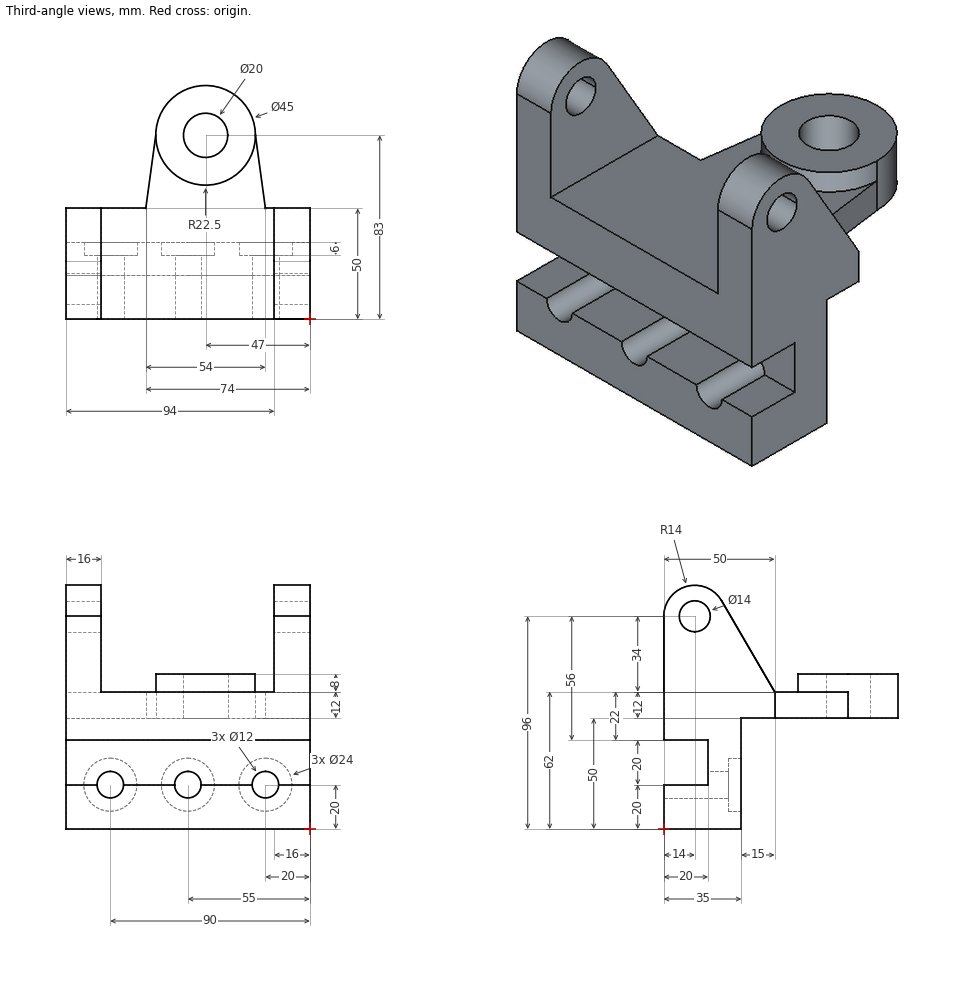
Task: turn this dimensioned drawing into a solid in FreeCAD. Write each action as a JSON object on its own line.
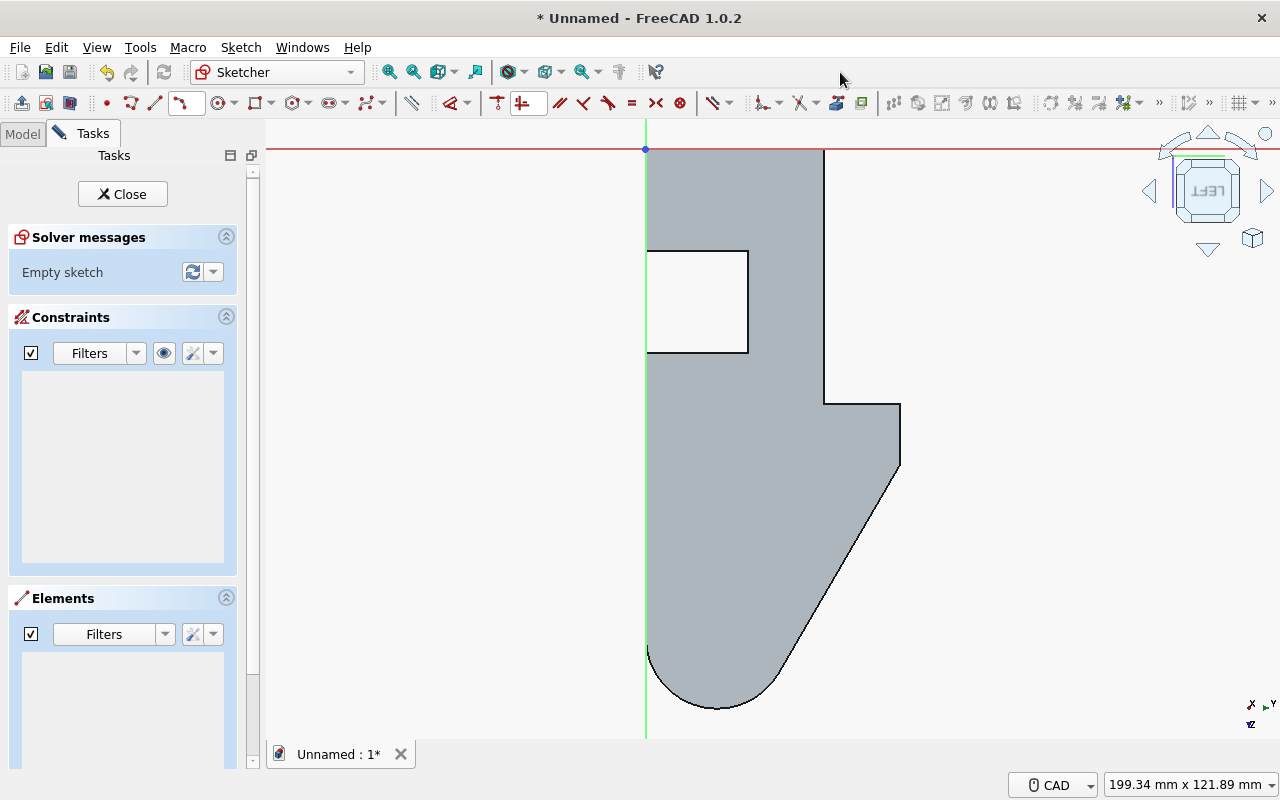
{"action": "scroll", "coordinate": [395, 711], "scroll_direction": "down", "scroll_amount": 1}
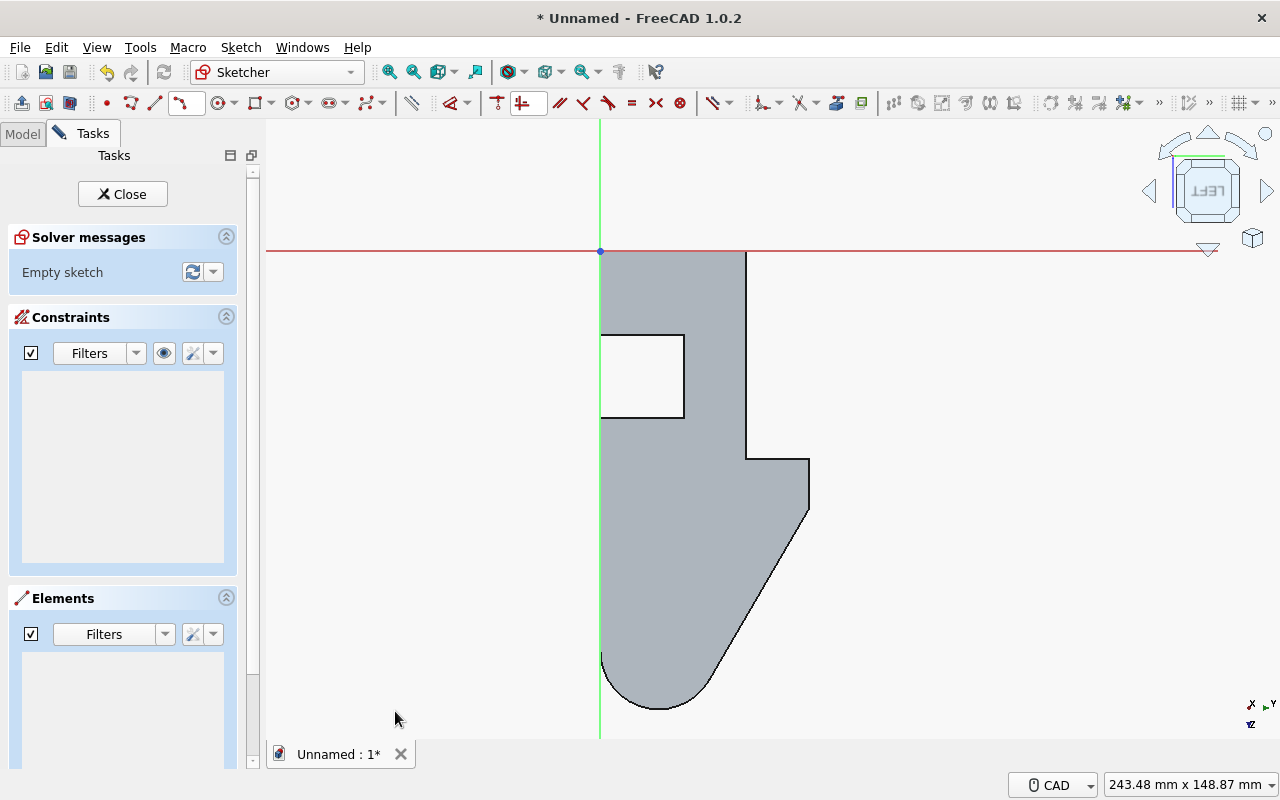
{"action": "scroll", "coordinate": [705, 281], "scroll_direction": "up", "scroll_amount": 2}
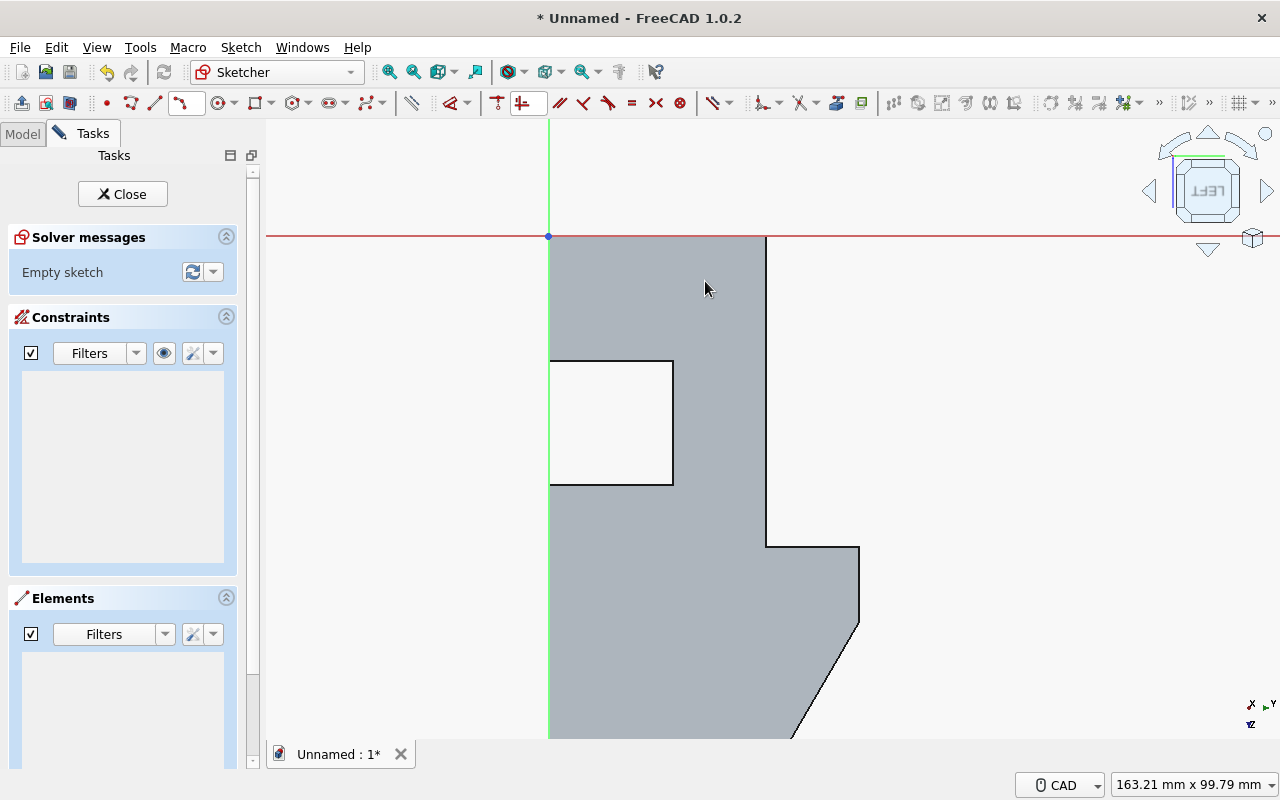
{"action": "key", "text": "g m"}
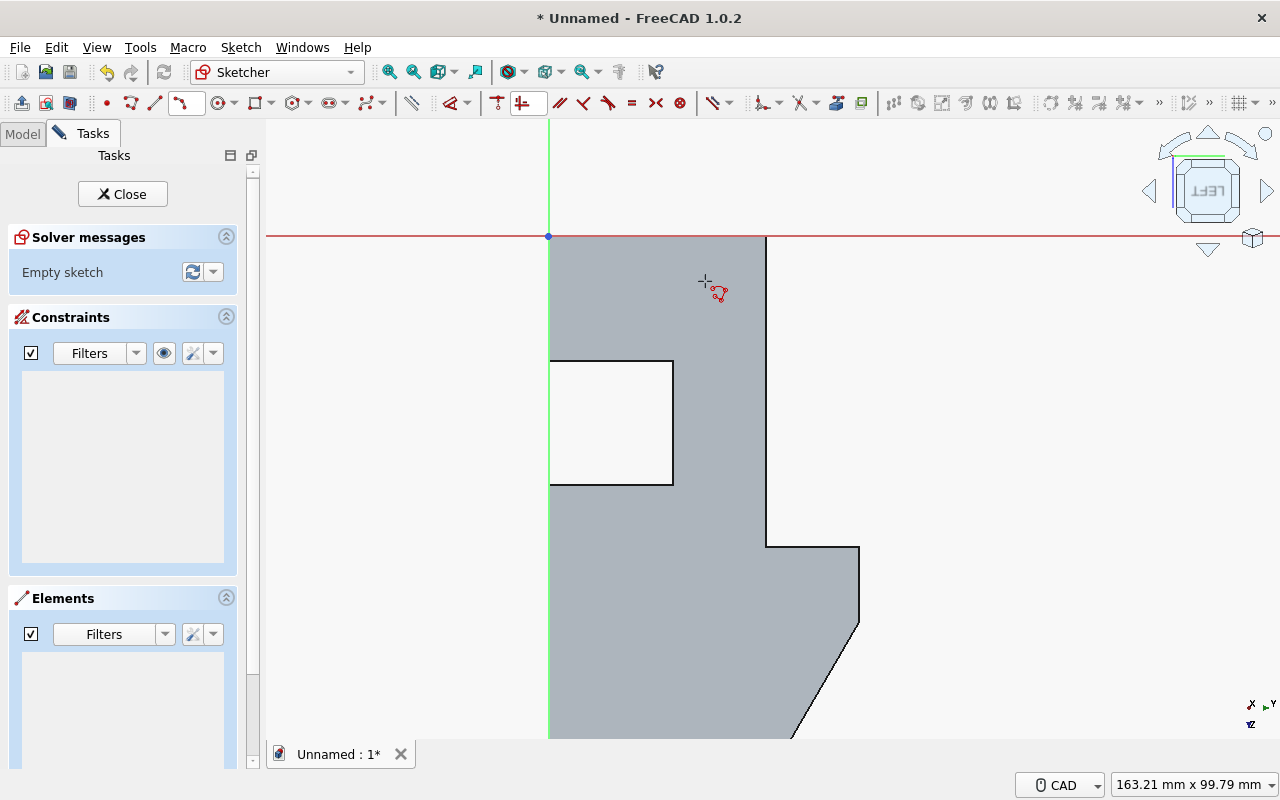
{"action": "left_click", "coordinate": [549, 236]}
{"action": "left_click", "coordinate": [558, 361]}
{"action": "left_click", "coordinate": [673, 361]}
{"action": "left_click", "coordinate": [673, 485]}
{"action": "left_click", "coordinate": [549, 485]}
{"action": "left_click", "coordinate": [558, 622]}
{"action": "left_click", "coordinate": [859, 622]}
{"action": "left_click", "coordinate": [859, 547]}
{"action": "left_click", "coordinate": [766, 547]}
{"action": "left_click", "coordinate": [766, 245]}
{"action": "left_click", "coordinate": [549, 236]}
{"action": "key", "text": "Escape"}
{"action": "key", "text": "Escape"}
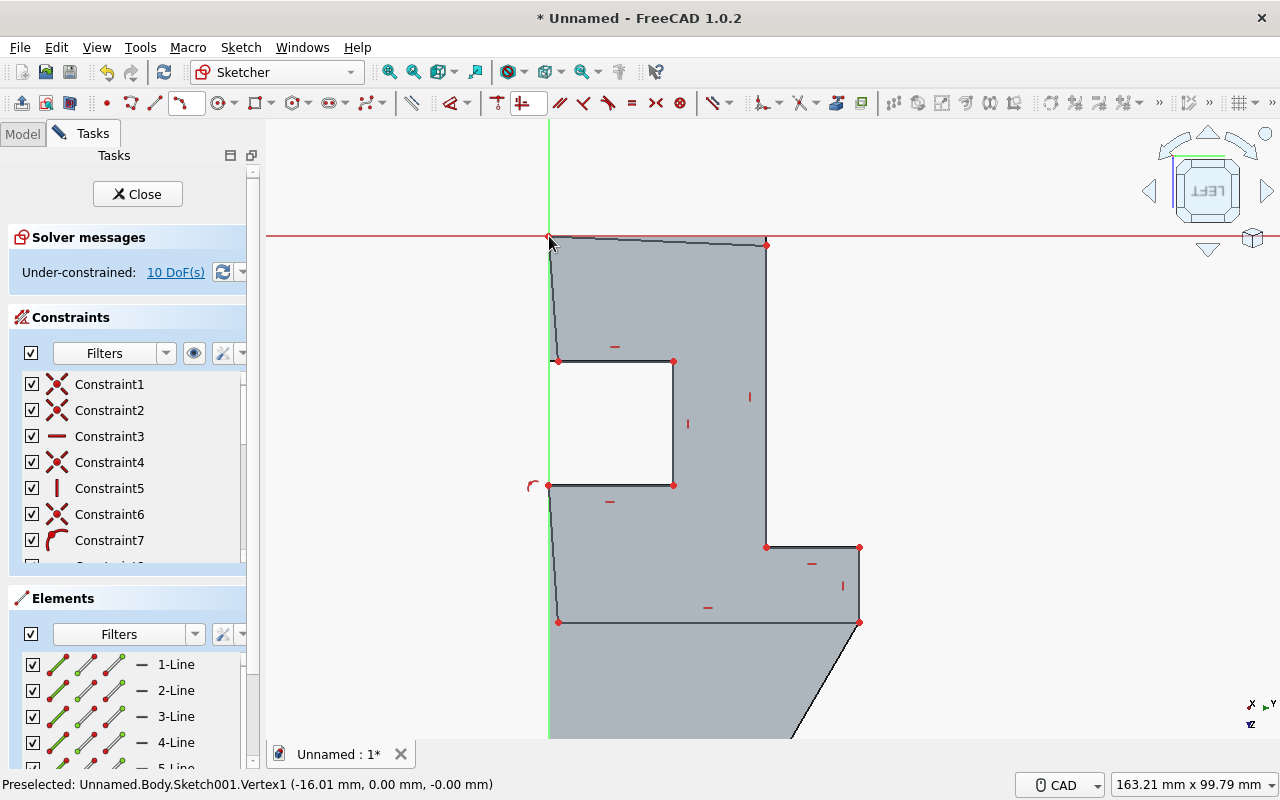
{"action": "left_click", "coordinate": [552, 274]}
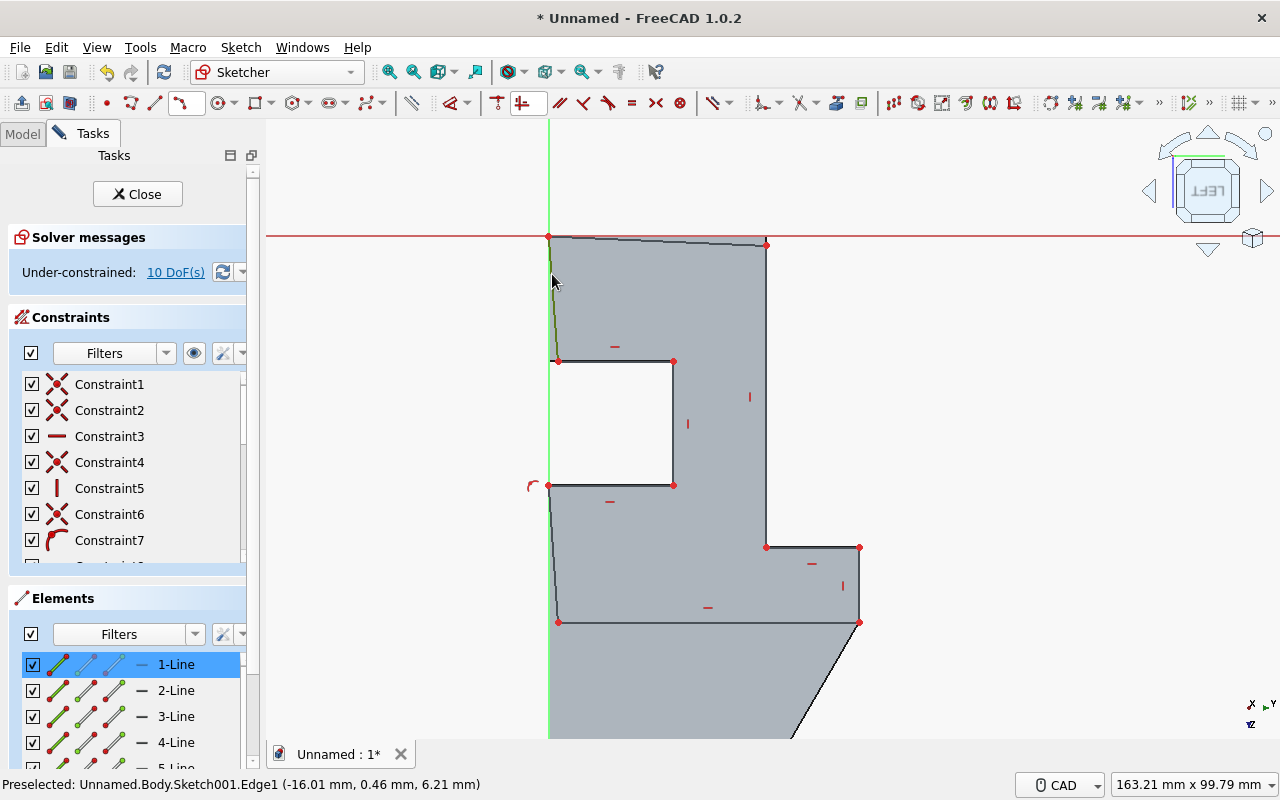
{"action": "left_click", "coordinate": [542, 104]}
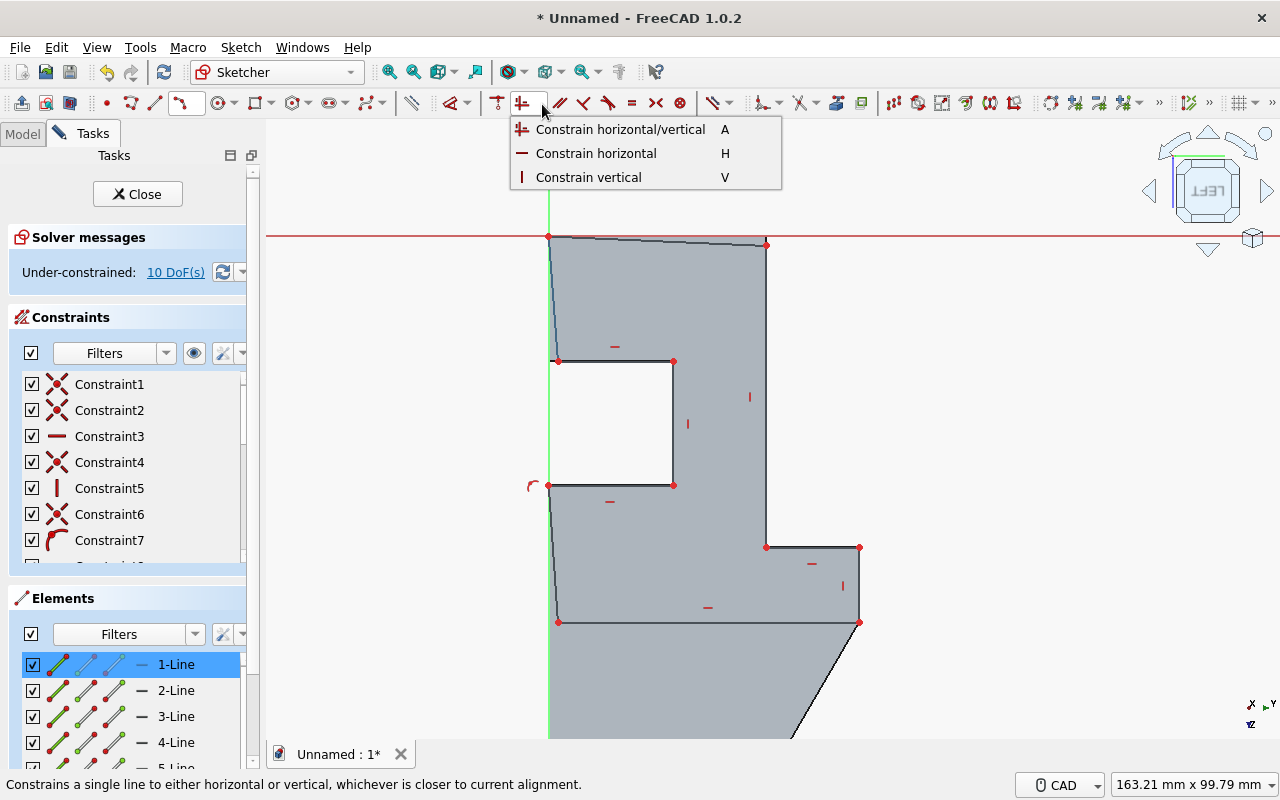
{"action": "left_click", "coordinate": [646, 177]}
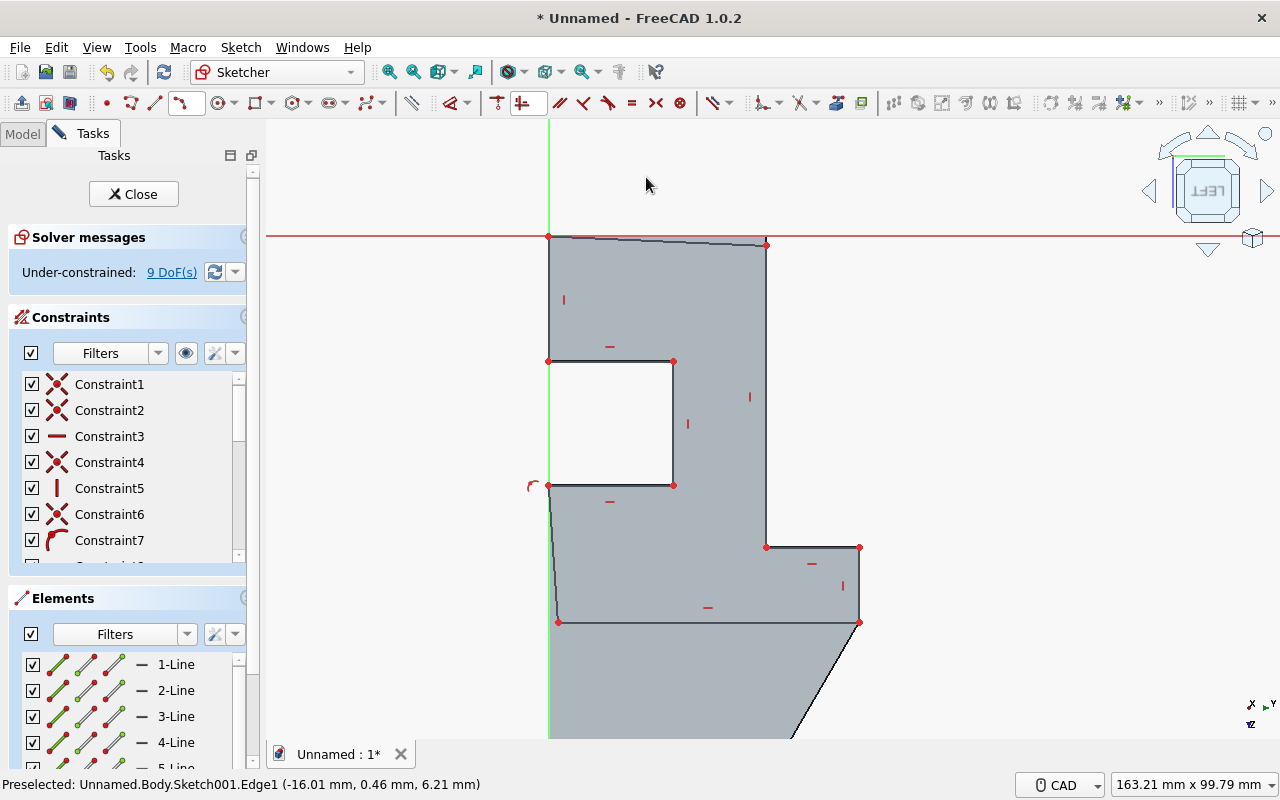
{"action": "left_click", "coordinate": [552, 527]}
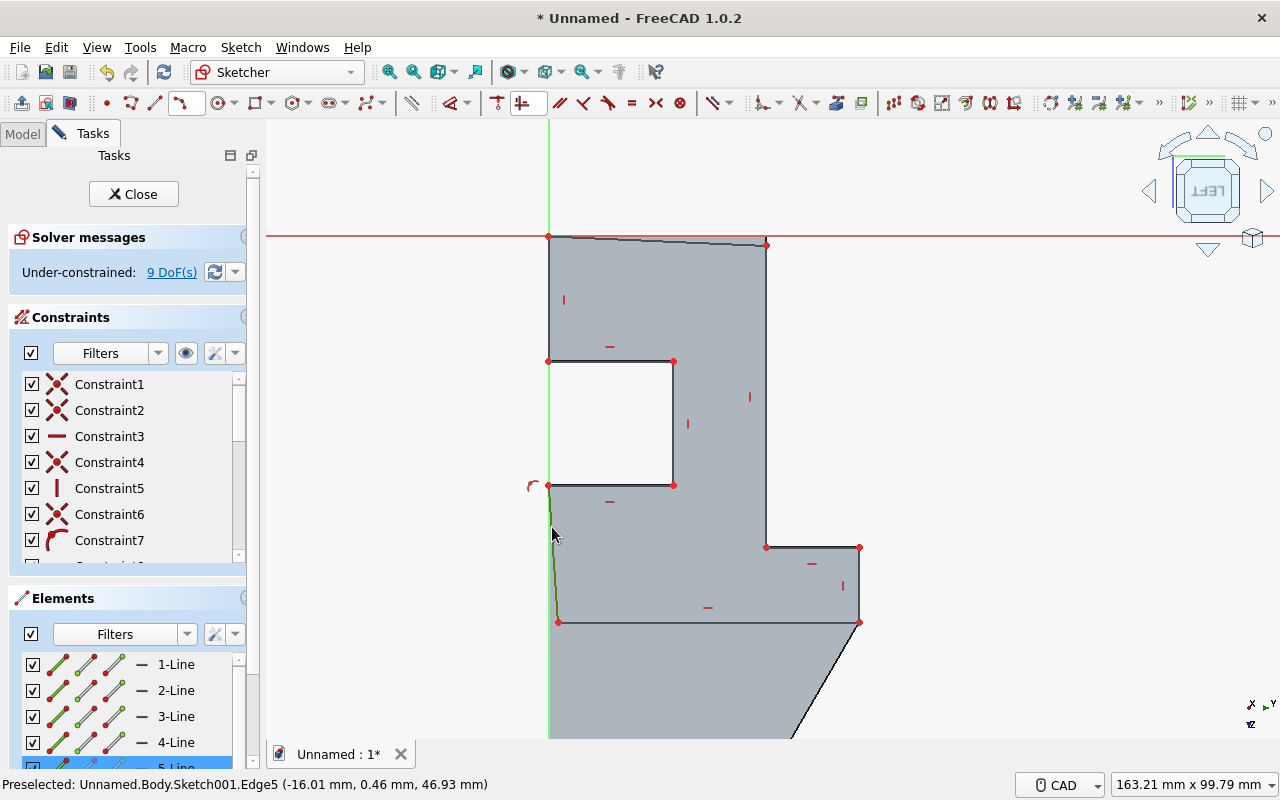
{"action": "key", "text": "v"}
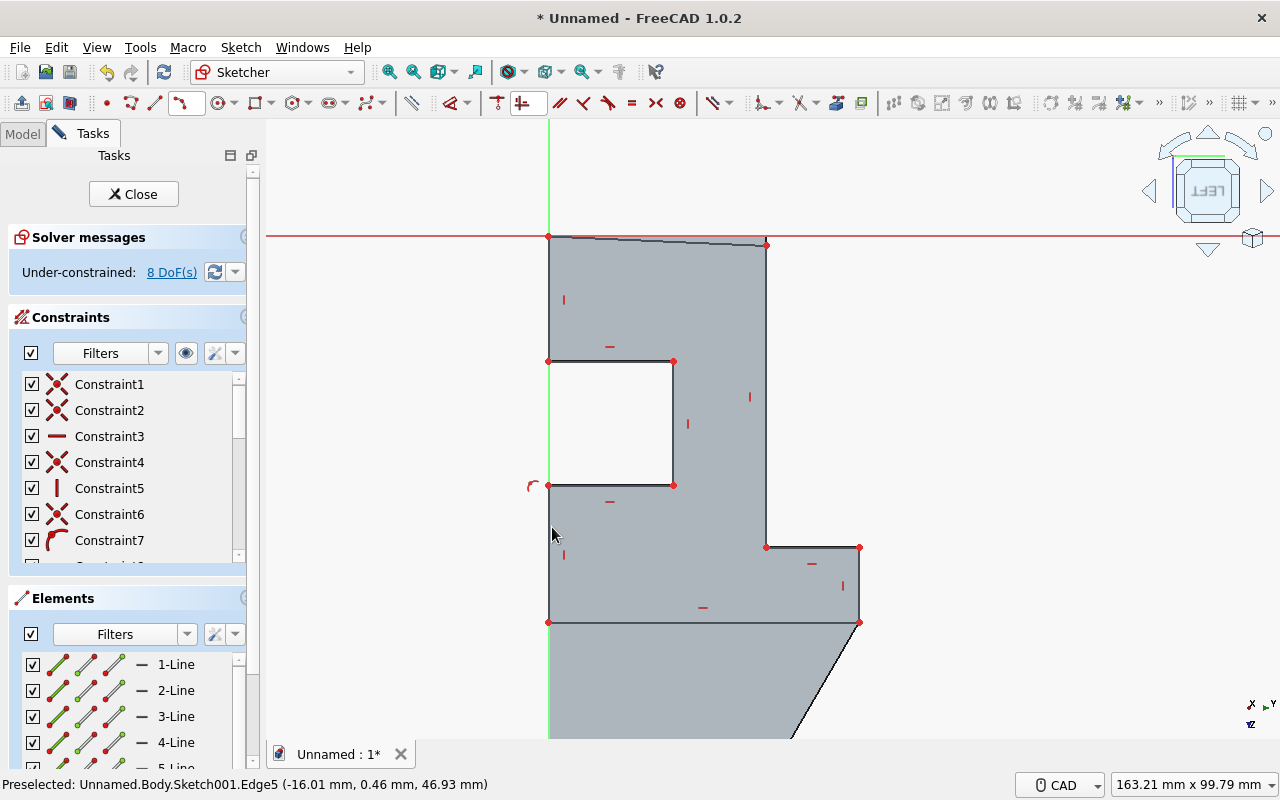
{"action": "left_click", "coordinate": [614, 239]}